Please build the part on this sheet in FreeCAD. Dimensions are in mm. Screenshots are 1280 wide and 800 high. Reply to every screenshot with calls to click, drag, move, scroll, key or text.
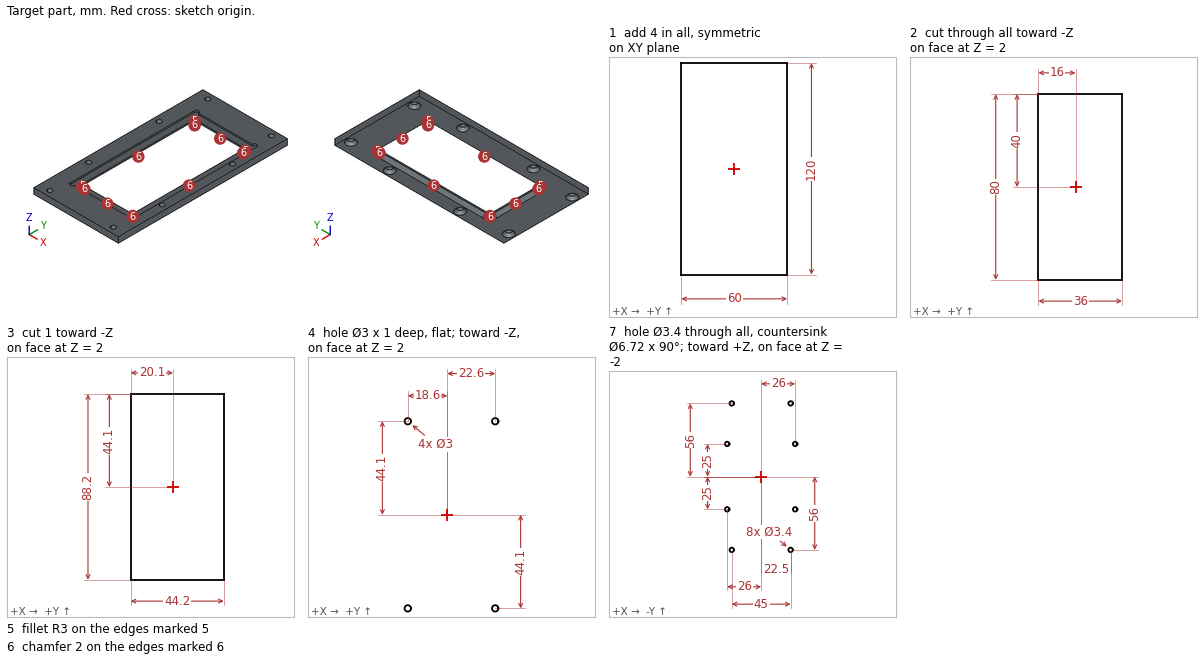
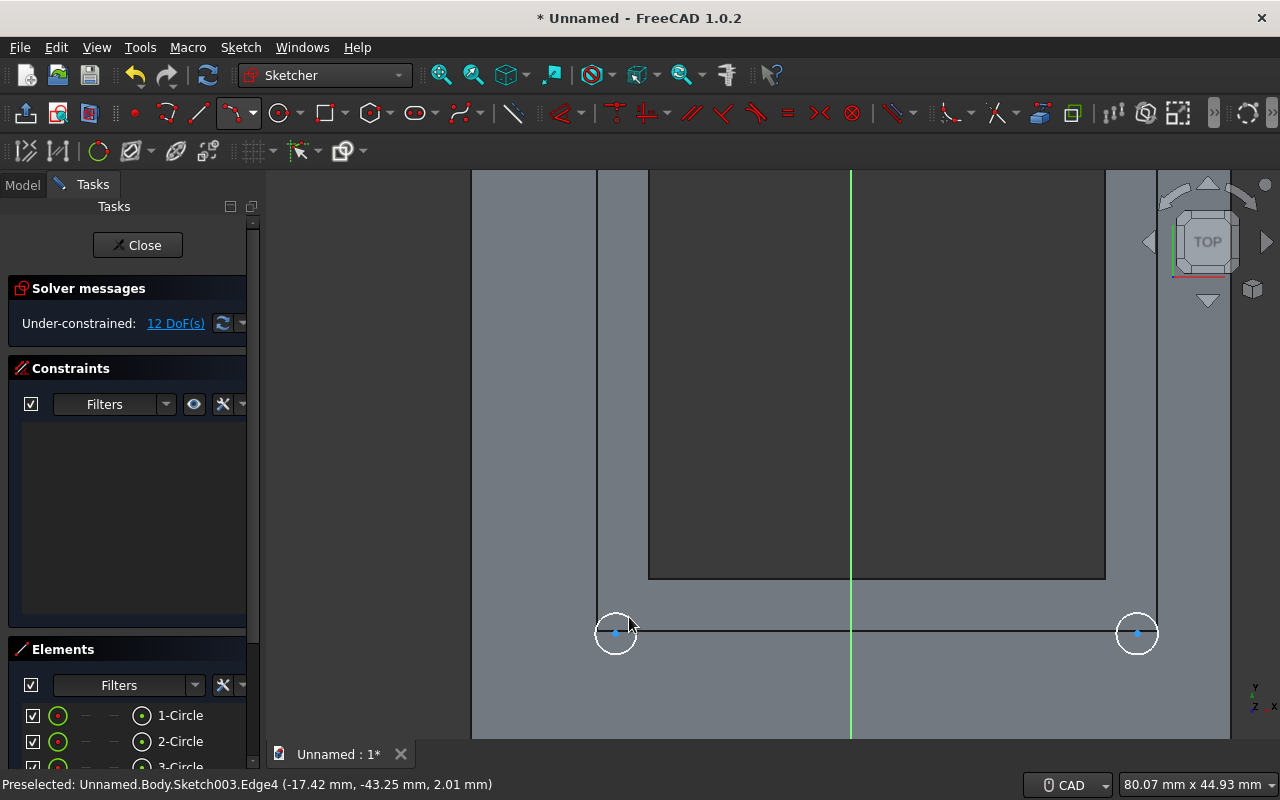
scroll(630, 619, down, 6)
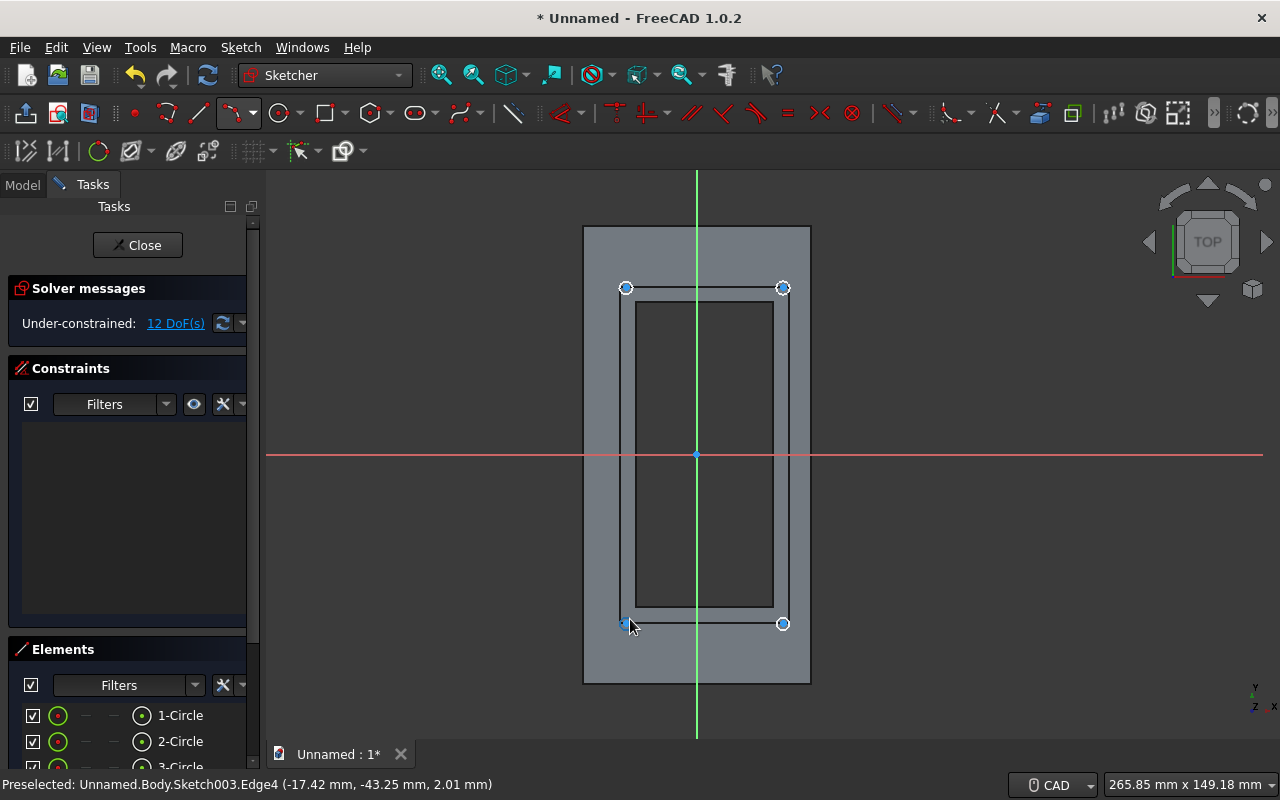
scroll(631, 283, up, 4)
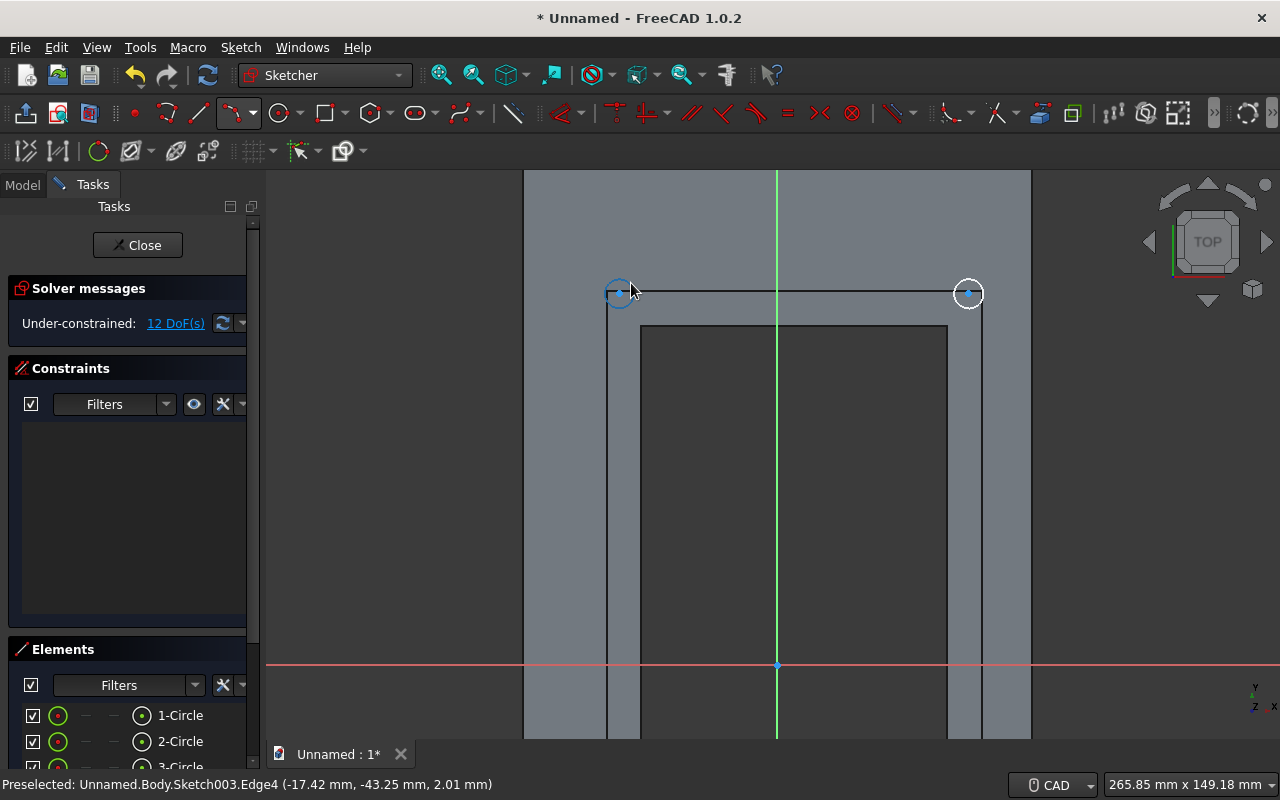
click(630, 284)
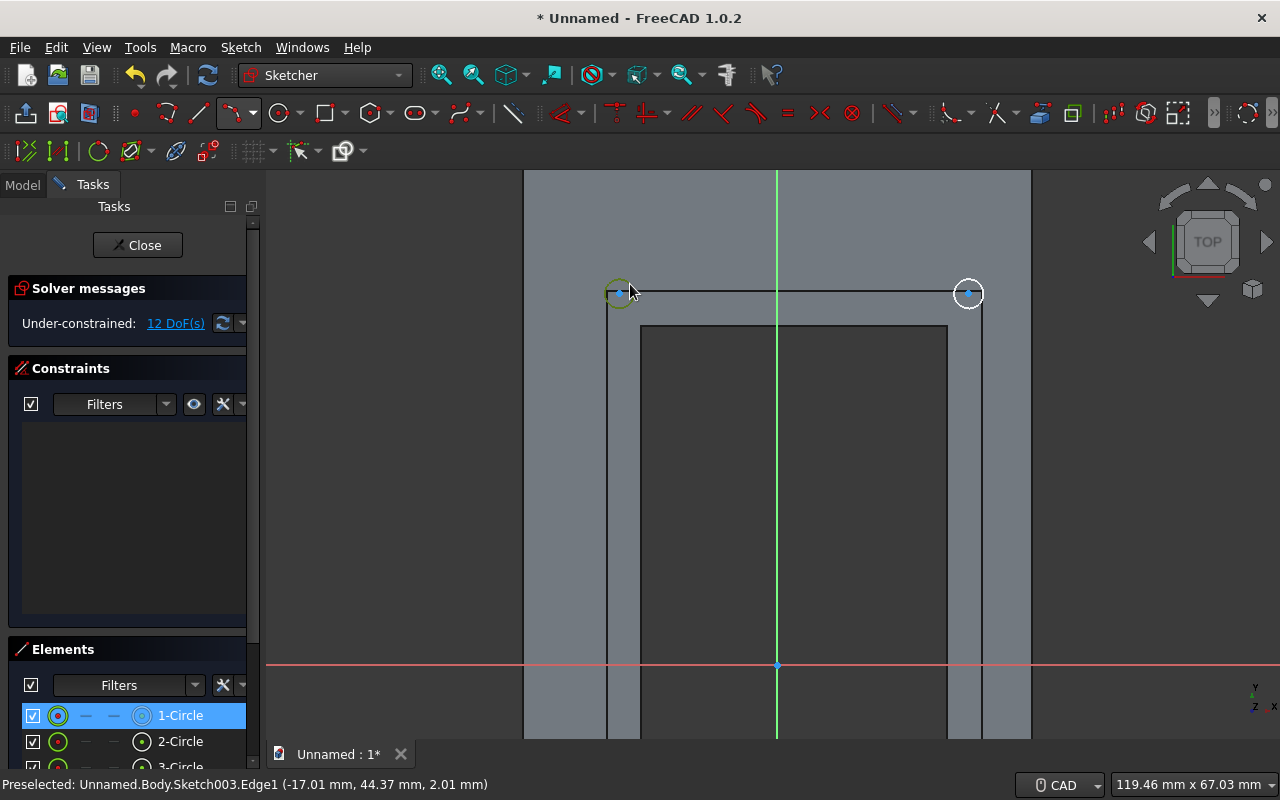
click(979, 284)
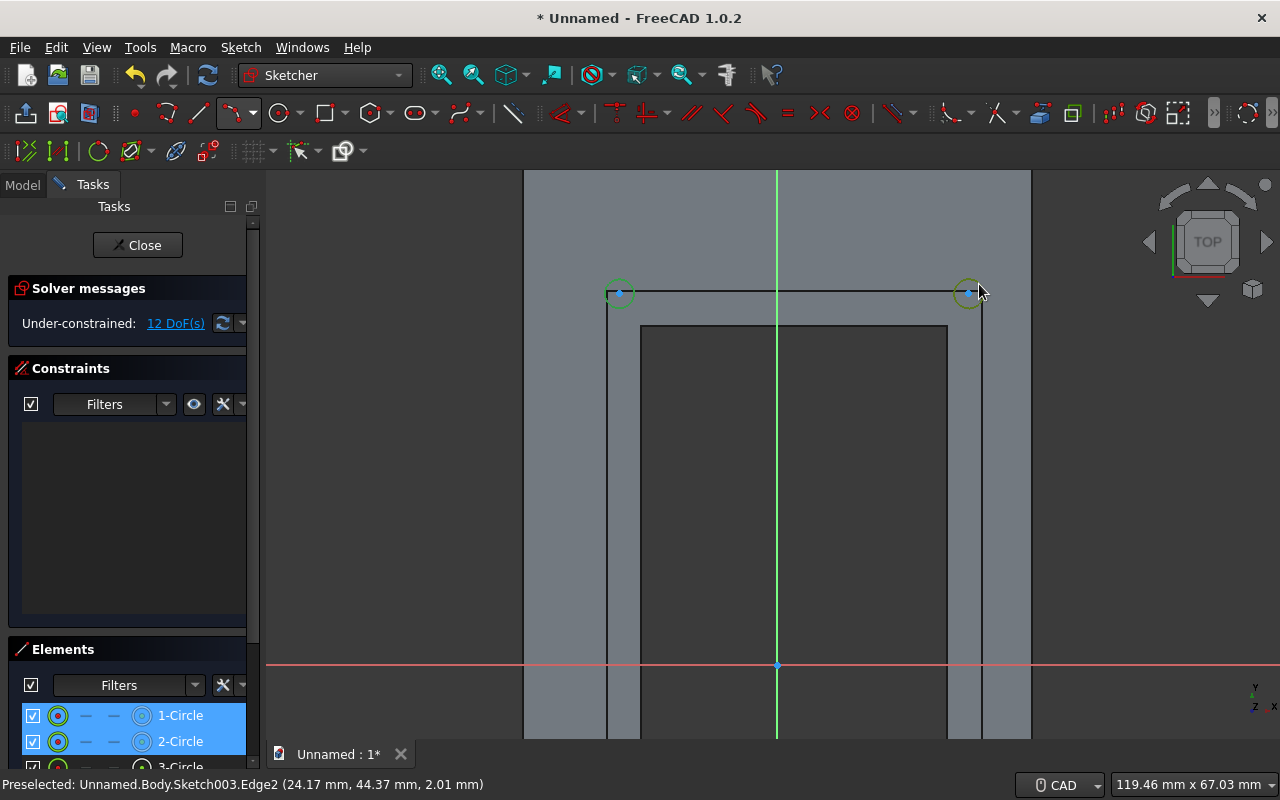
scroll(631, 283, down, 4)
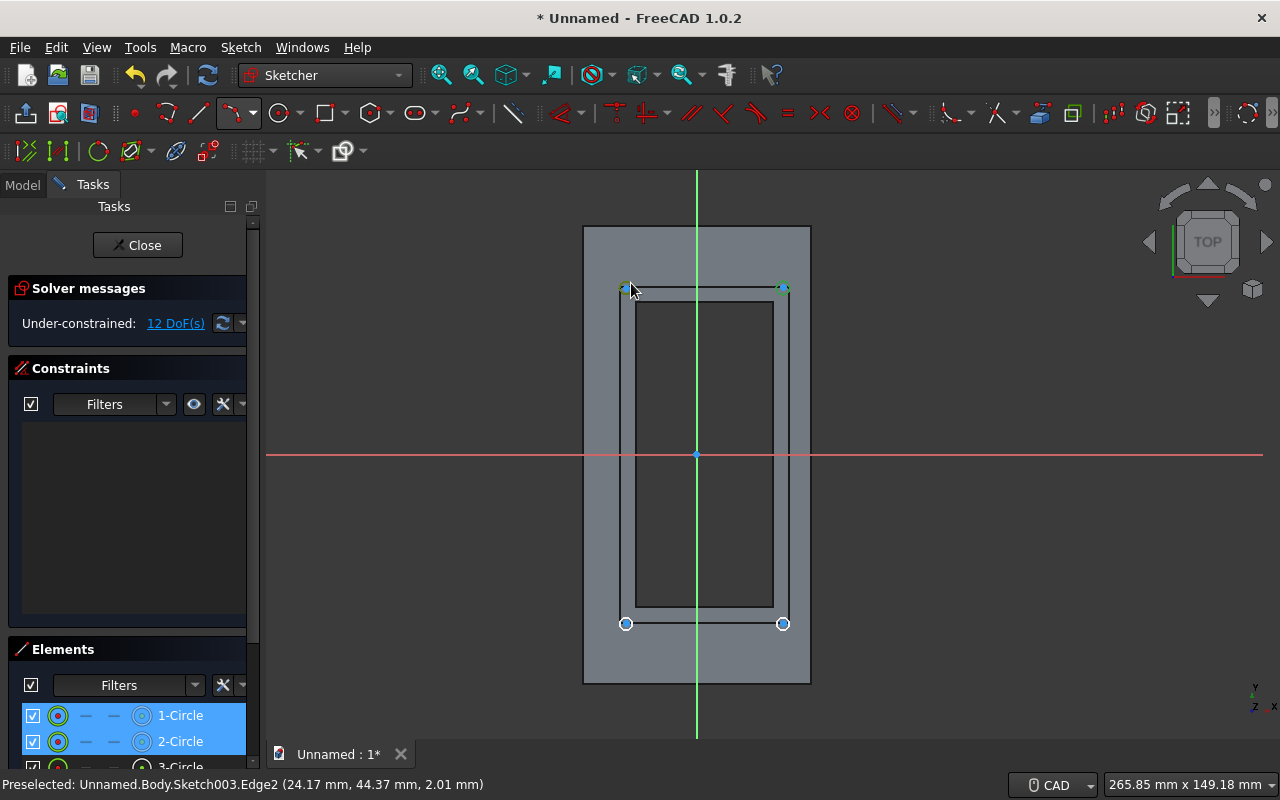
scroll(787, 620, up, 4)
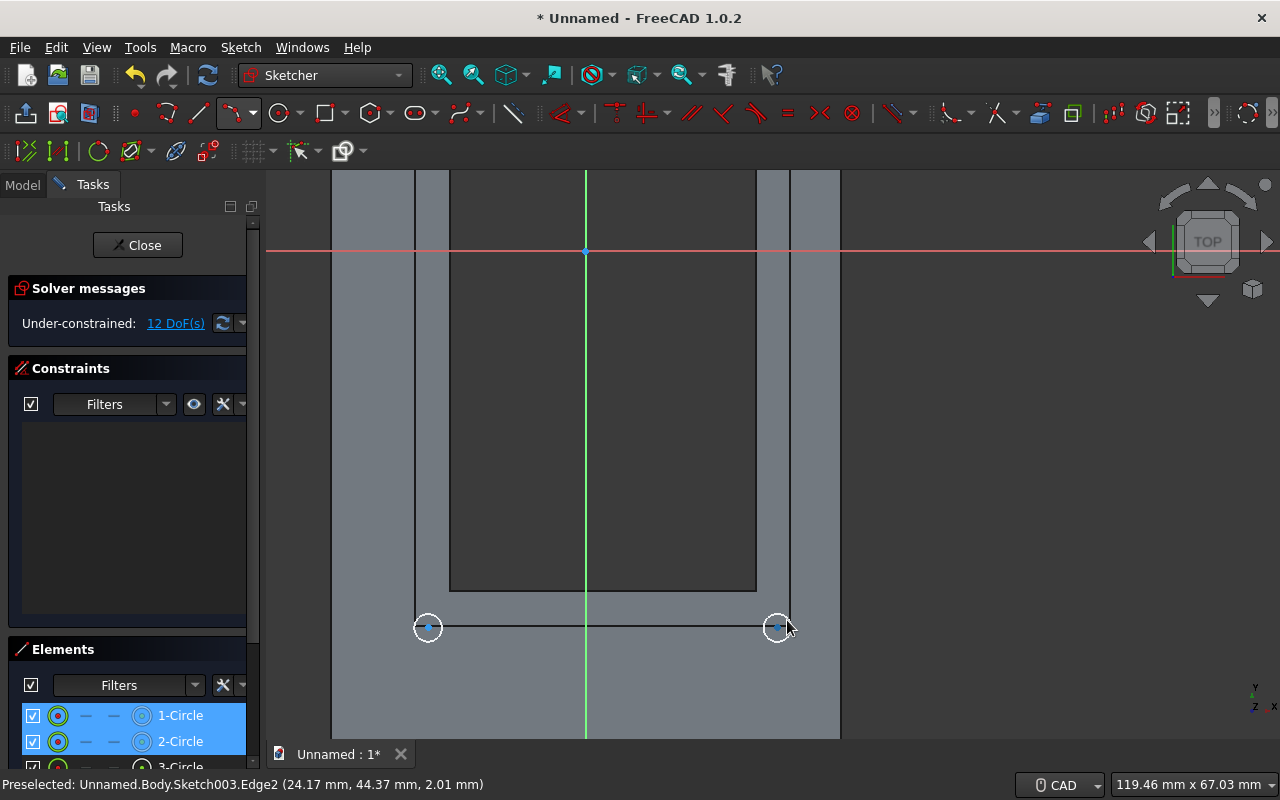
click(787, 618)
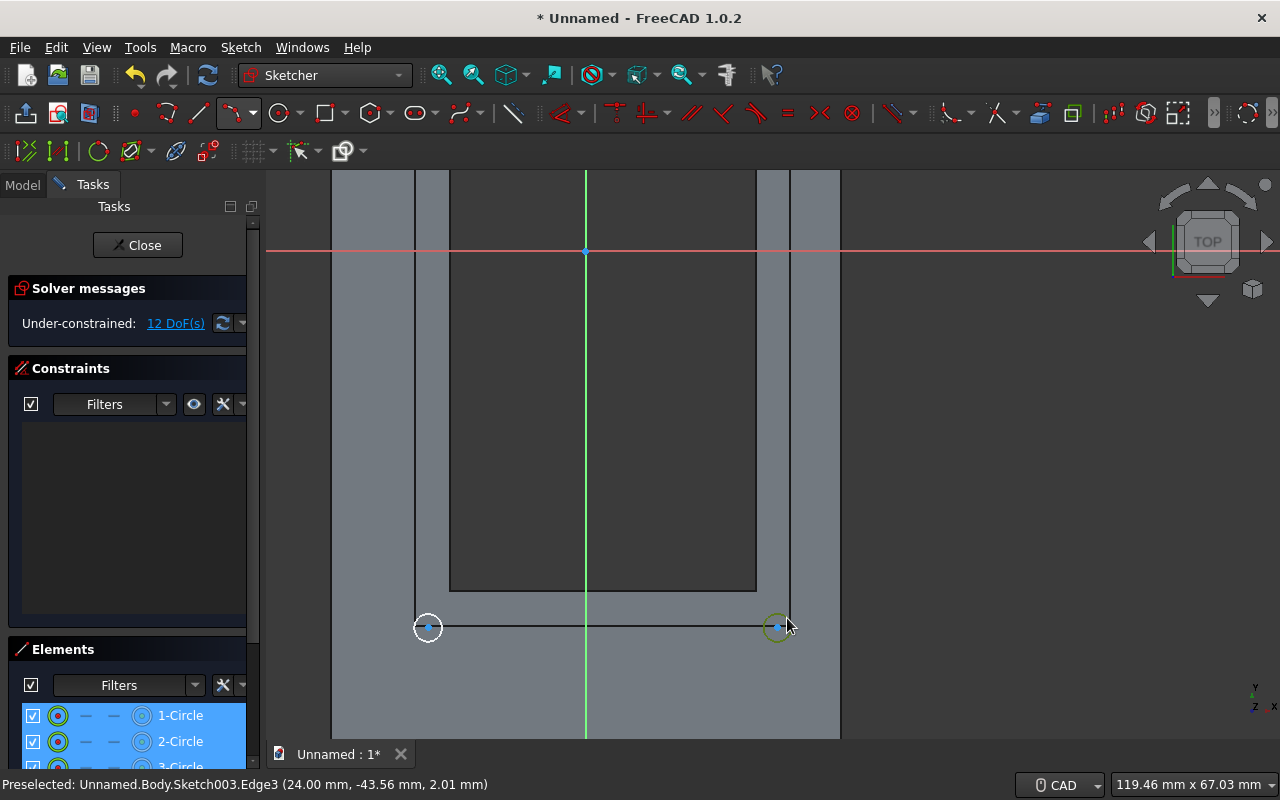
click(438, 618)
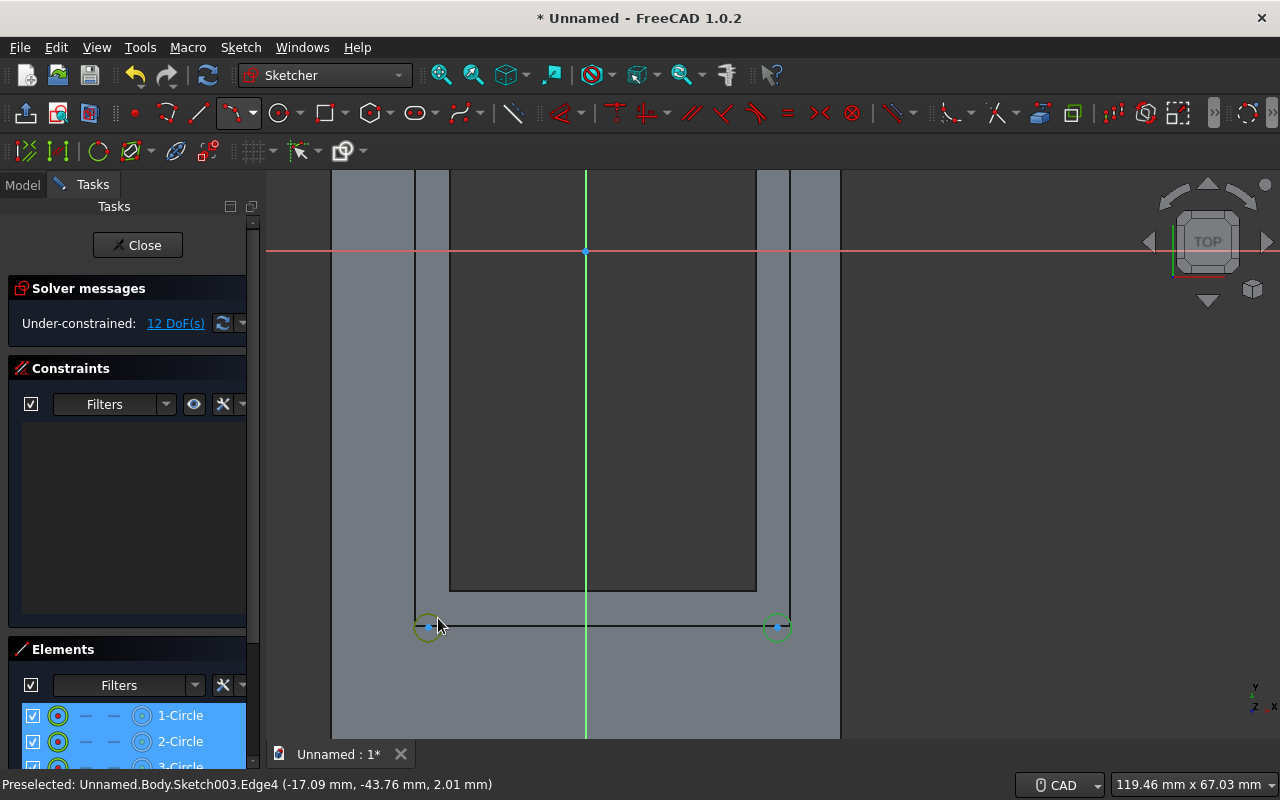
click(788, 114)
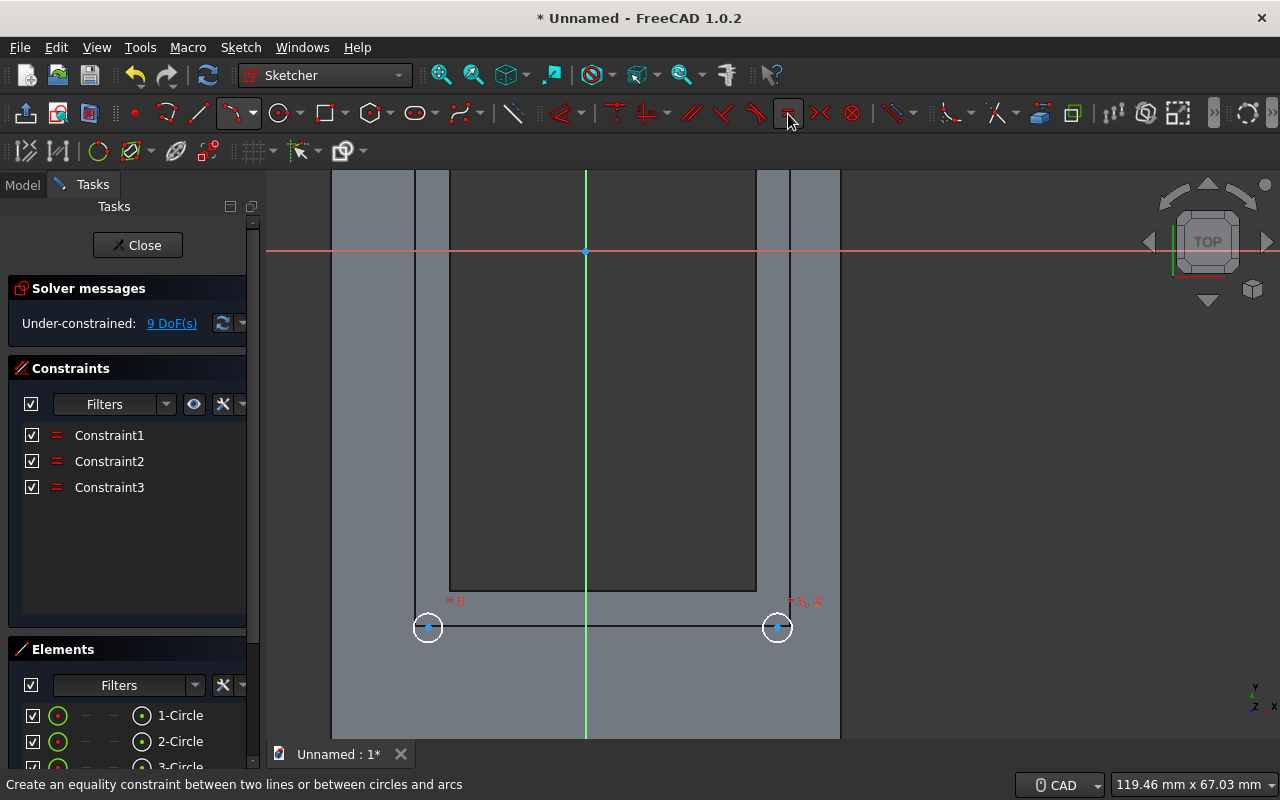
scroll(787, 620, down, 4)